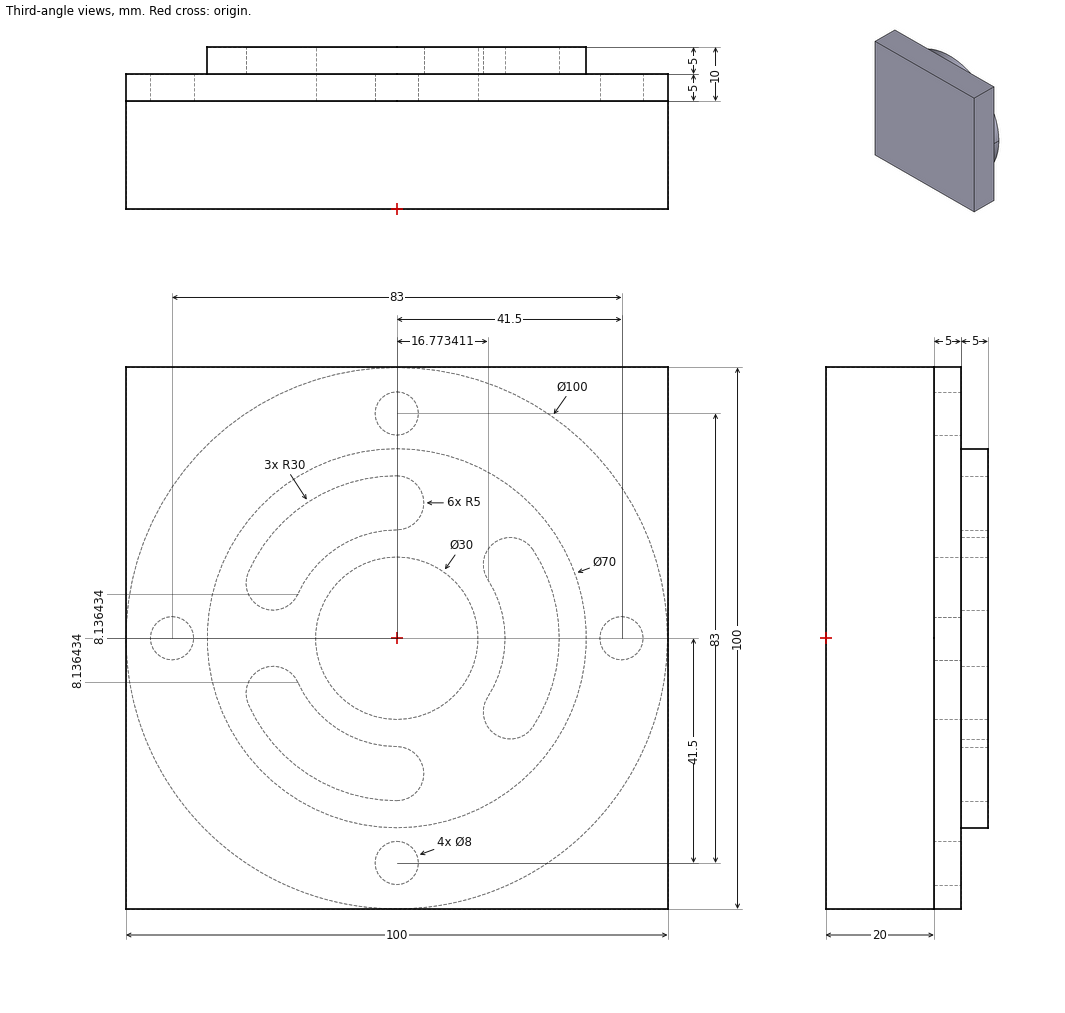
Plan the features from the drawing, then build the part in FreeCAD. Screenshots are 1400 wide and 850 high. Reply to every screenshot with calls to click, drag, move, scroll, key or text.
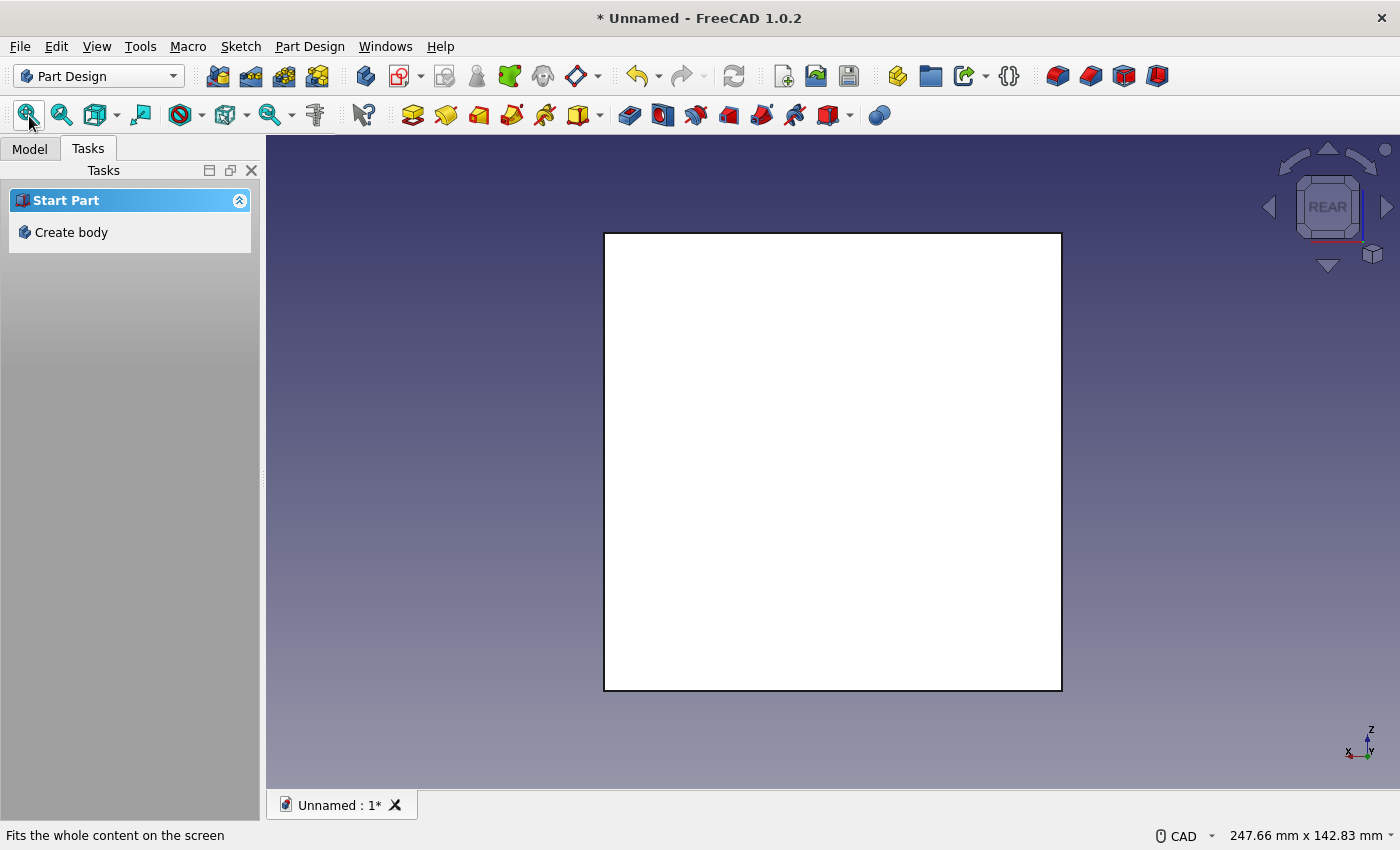
click(833, 461)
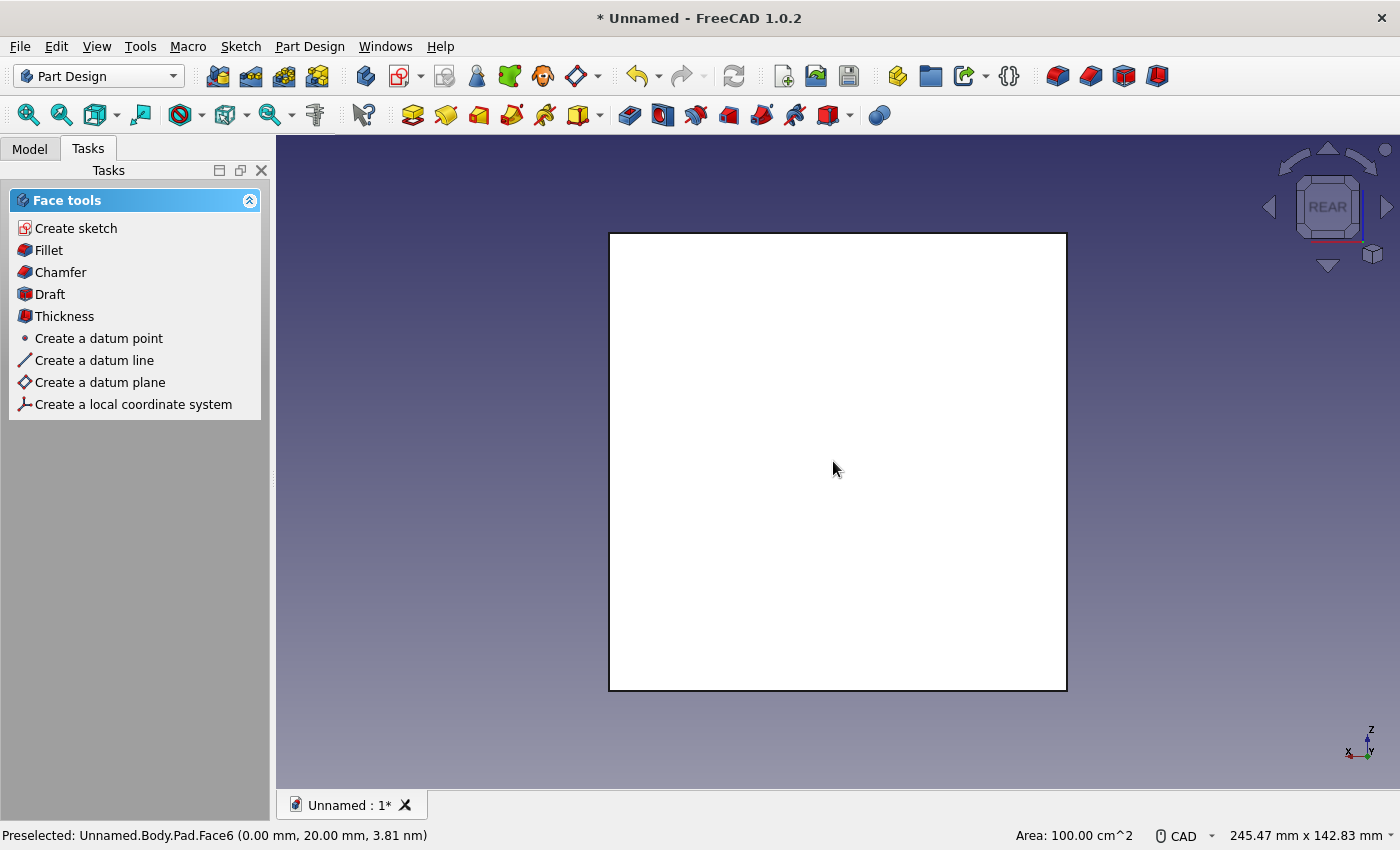
click(398, 76)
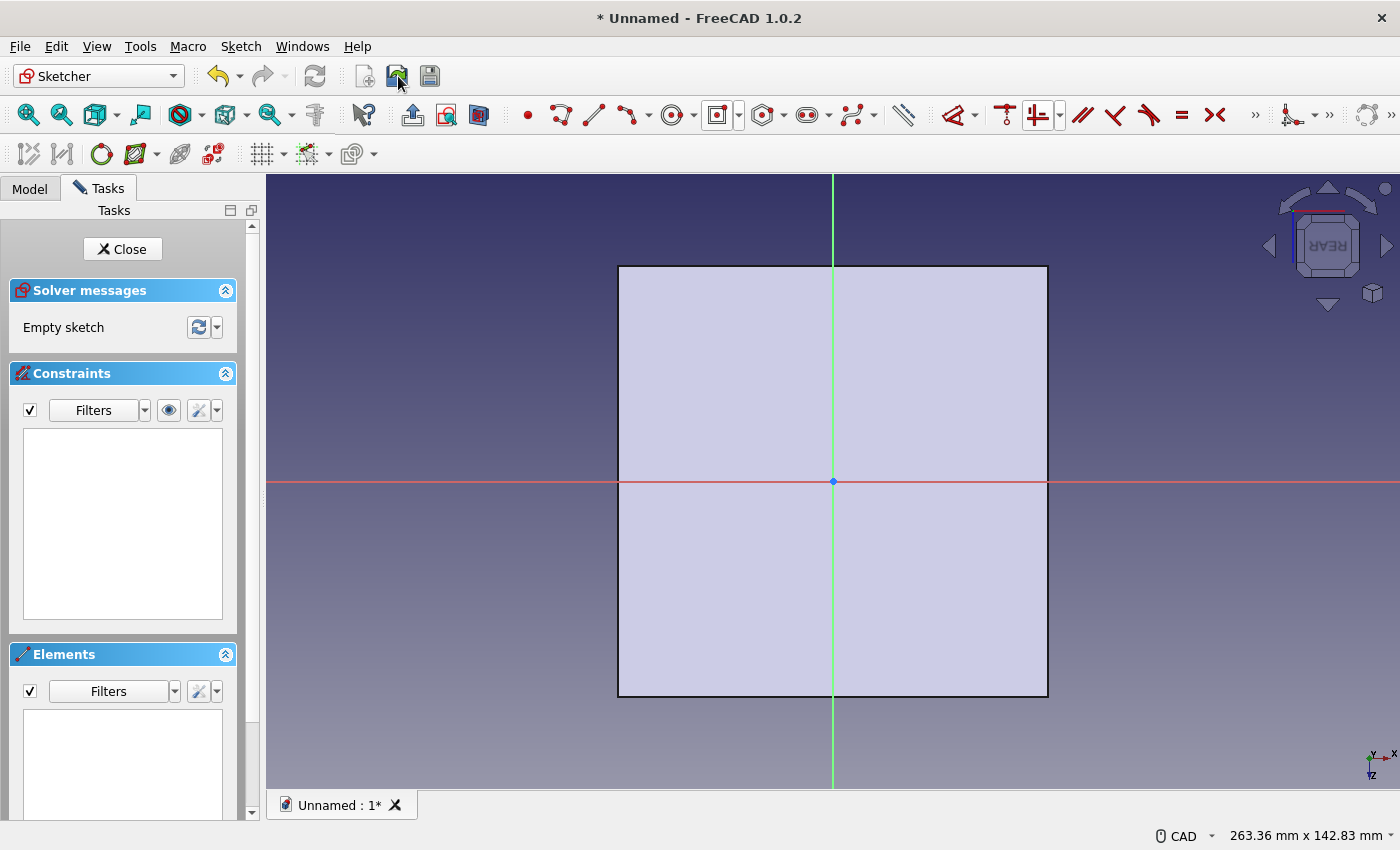
click(672, 116)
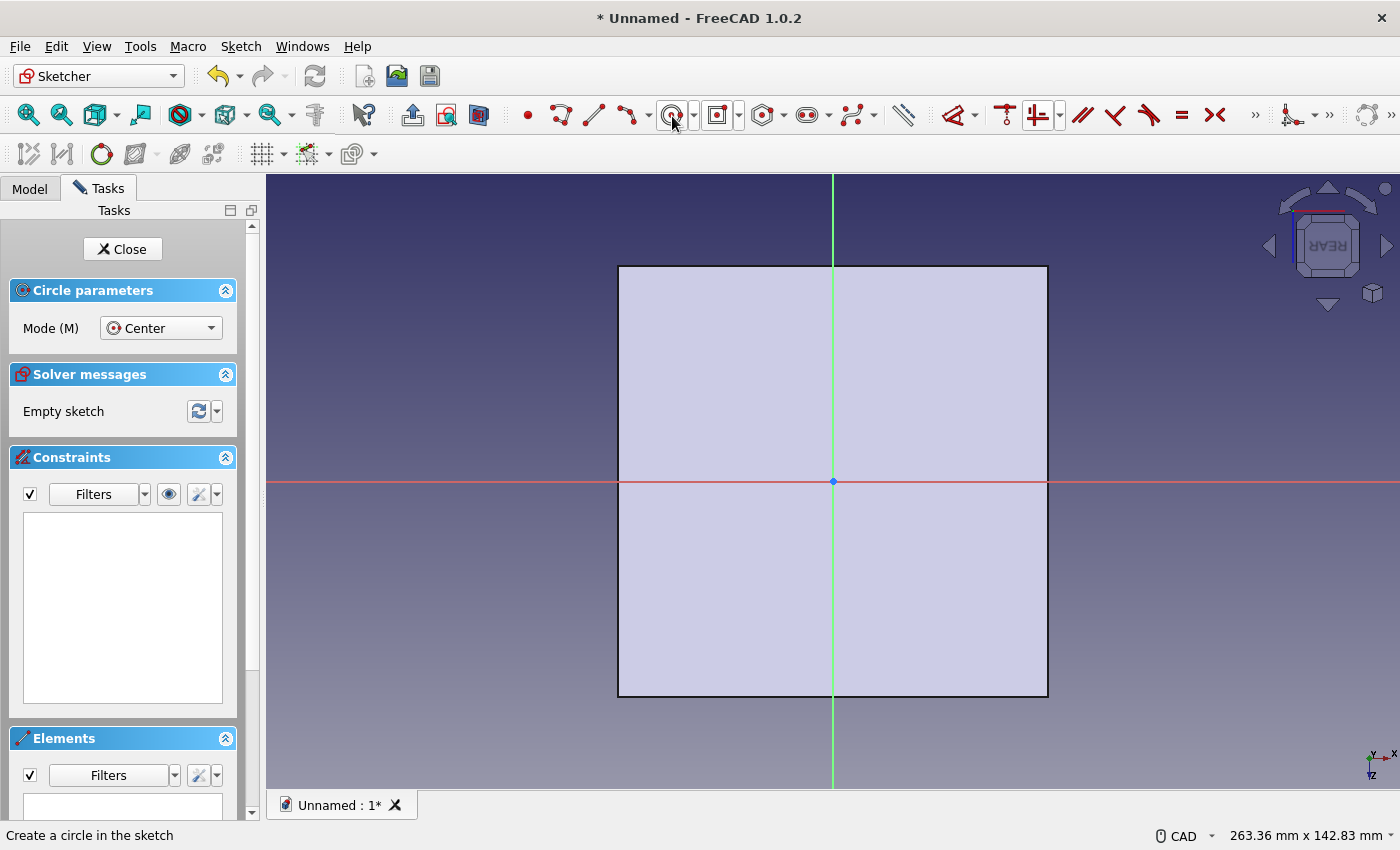
click(833, 482)
move(985, 329)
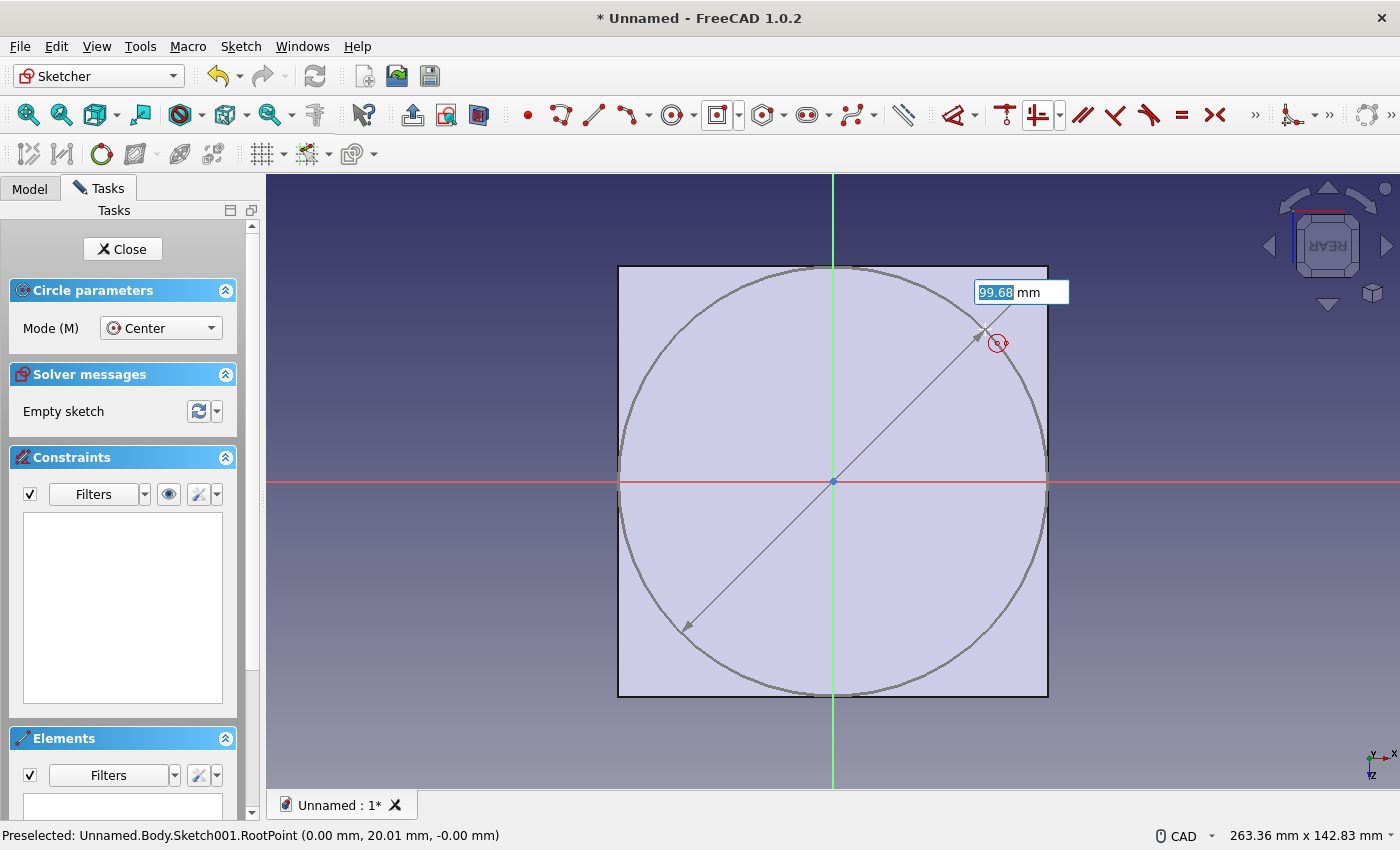
text(100)
key(Return)
key(Escape)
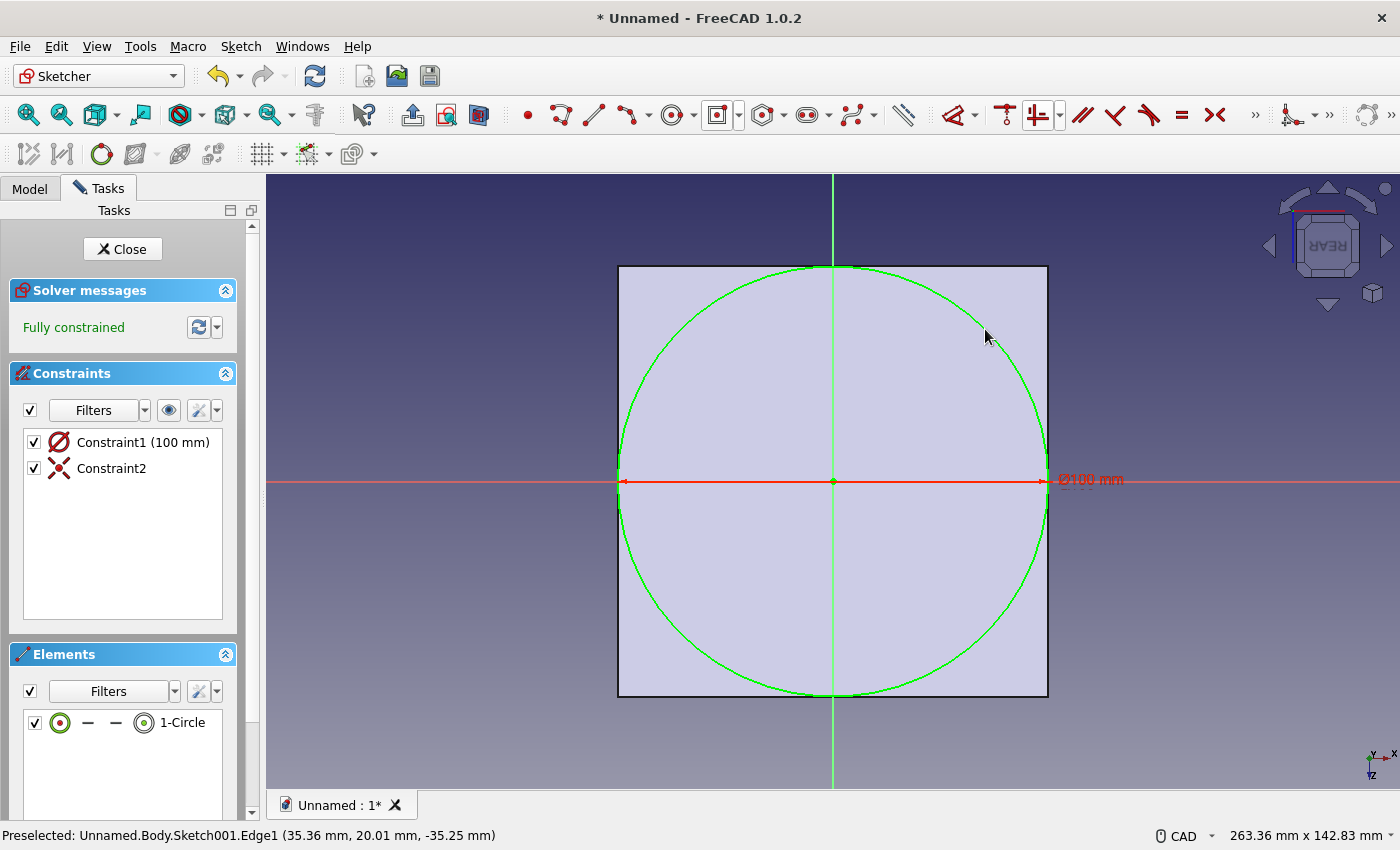
click(123, 249)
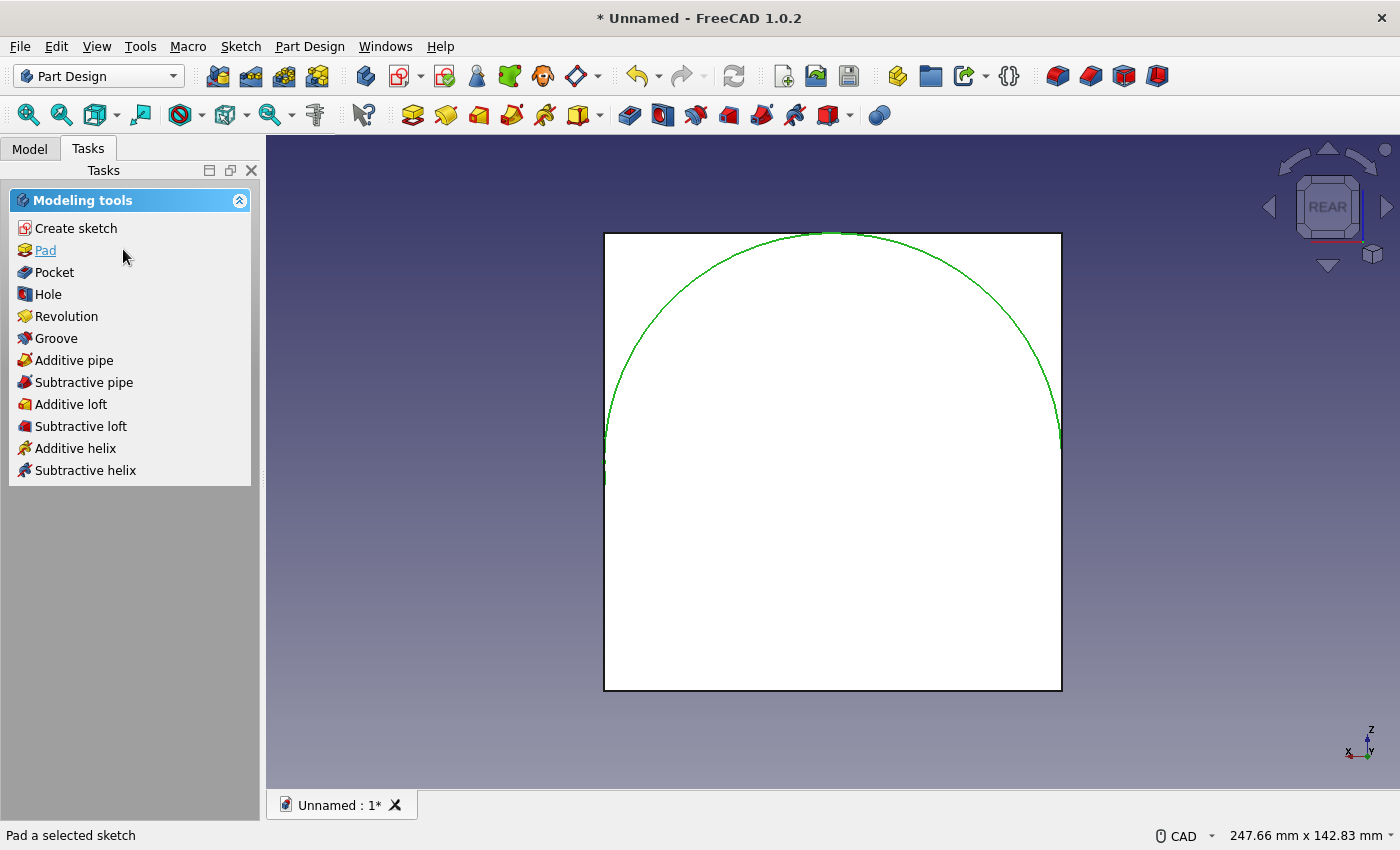
click(413, 116)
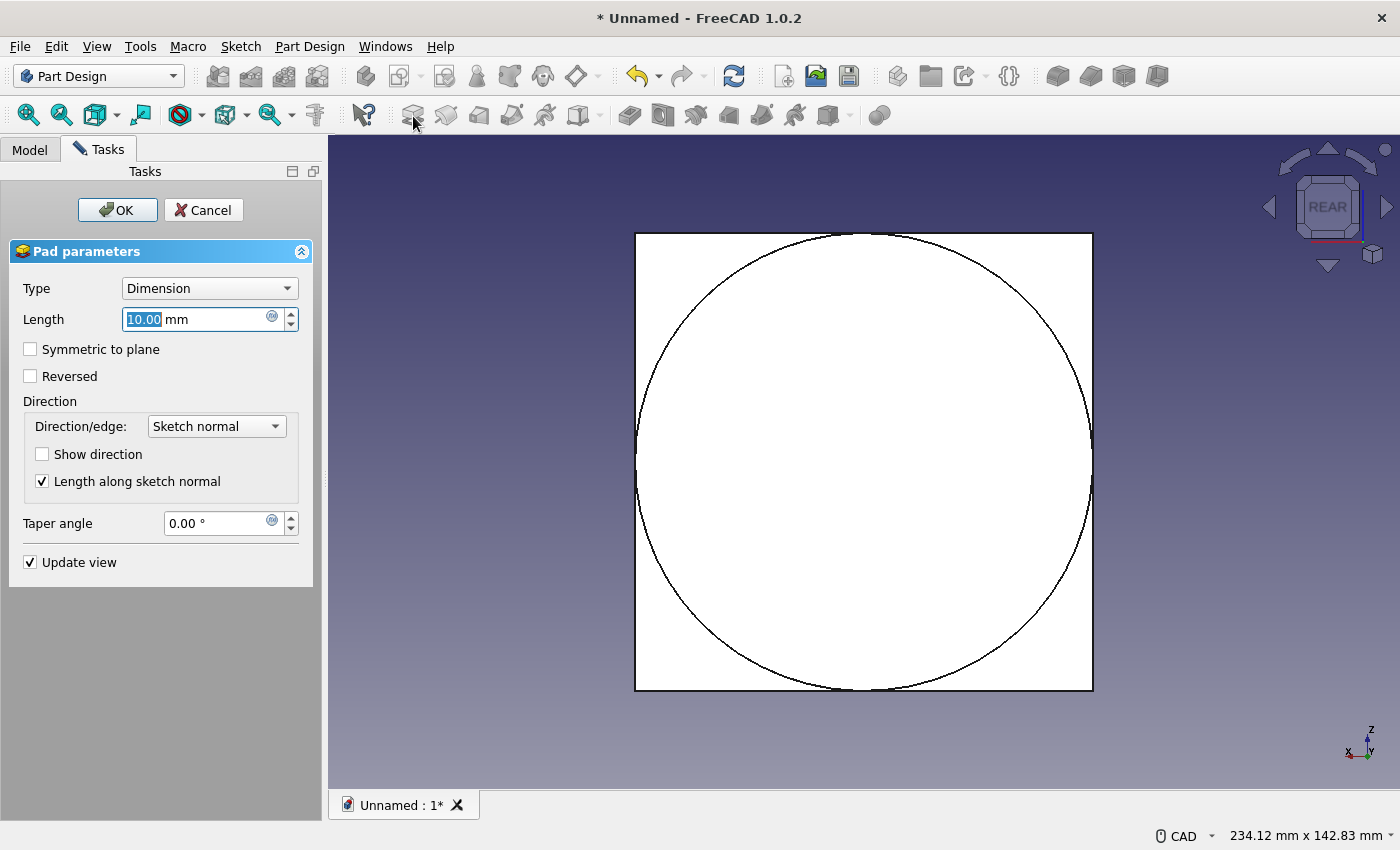
text(5)
key(Tab)